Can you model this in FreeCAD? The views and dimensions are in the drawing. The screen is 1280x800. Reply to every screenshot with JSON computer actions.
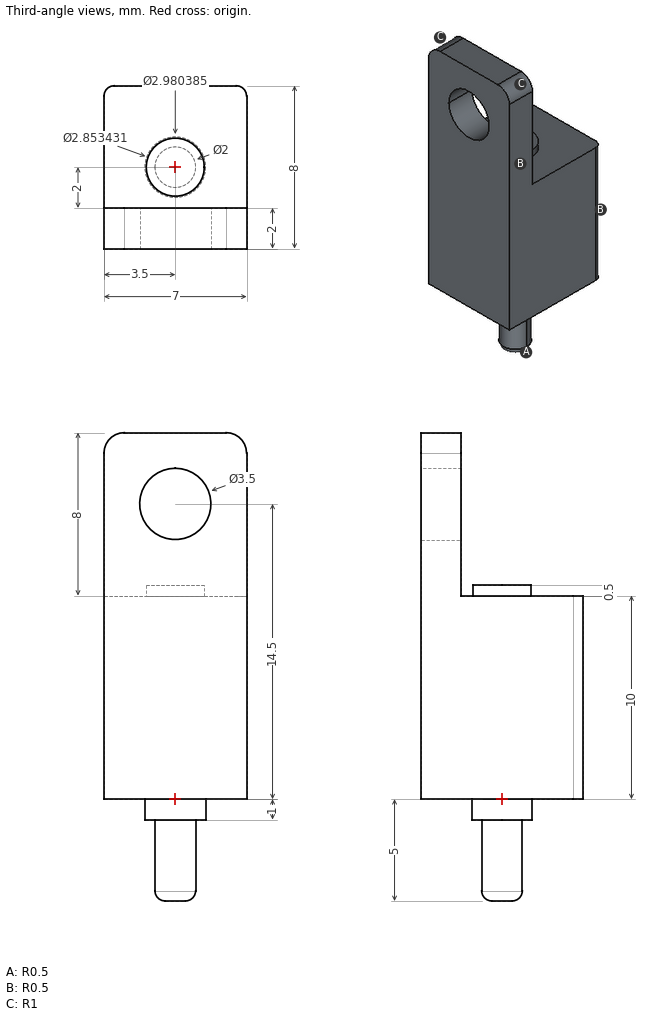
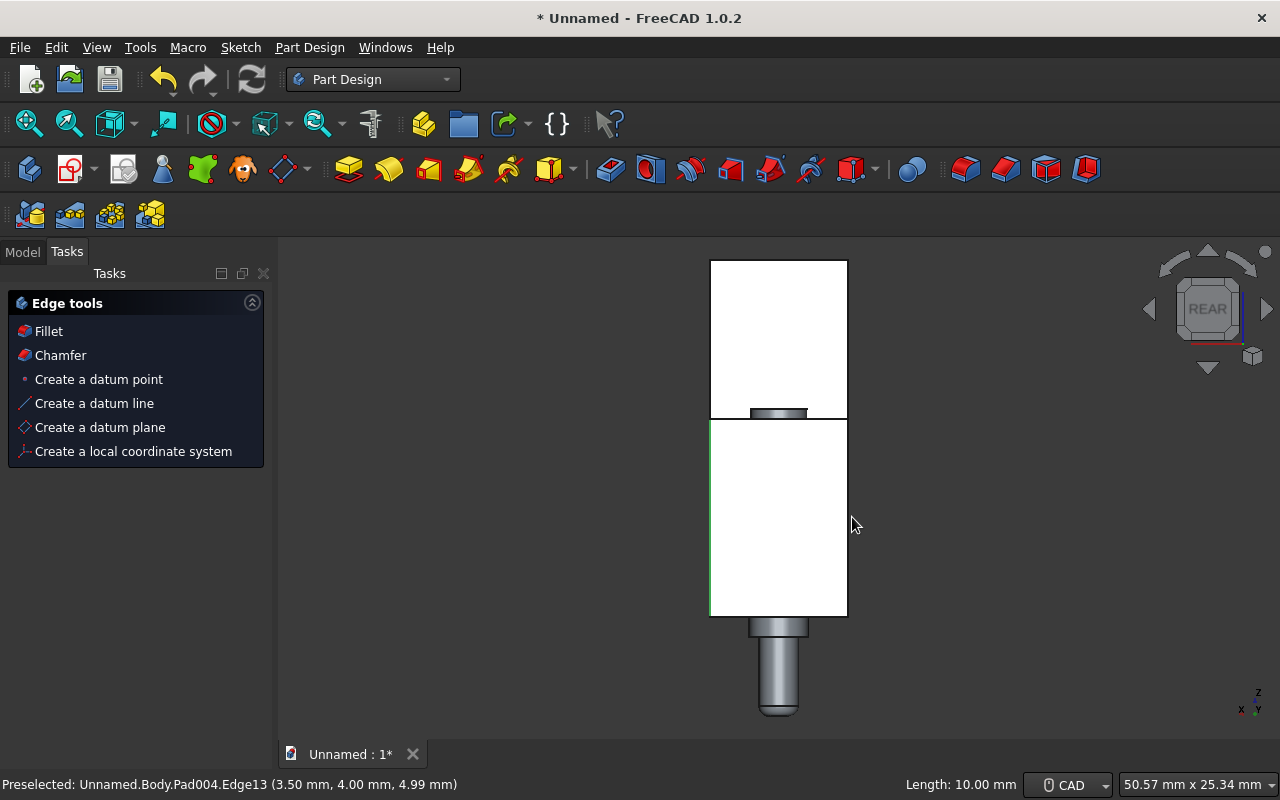
{"action": "left_click", "coordinate": [848, 517], "text": "ctrl"}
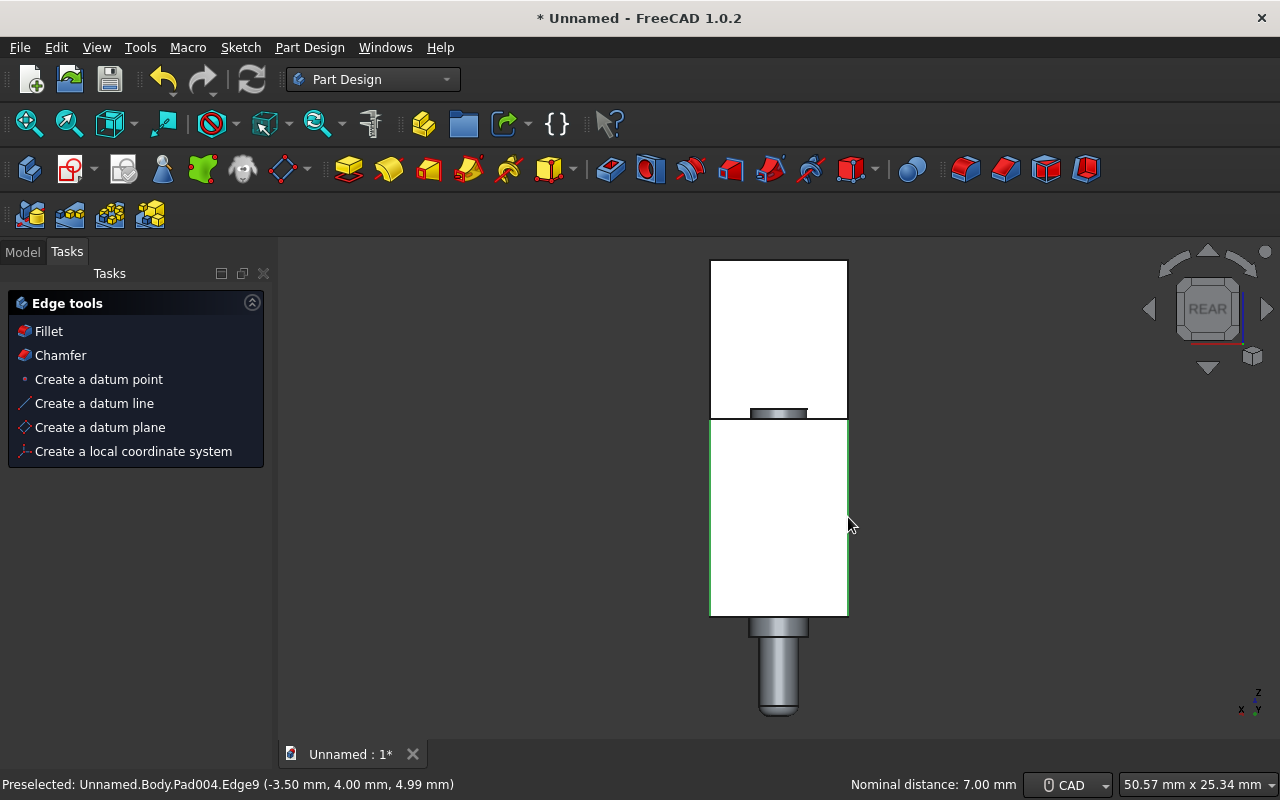
{"action": "left_click", "coordinate": [966, 170]}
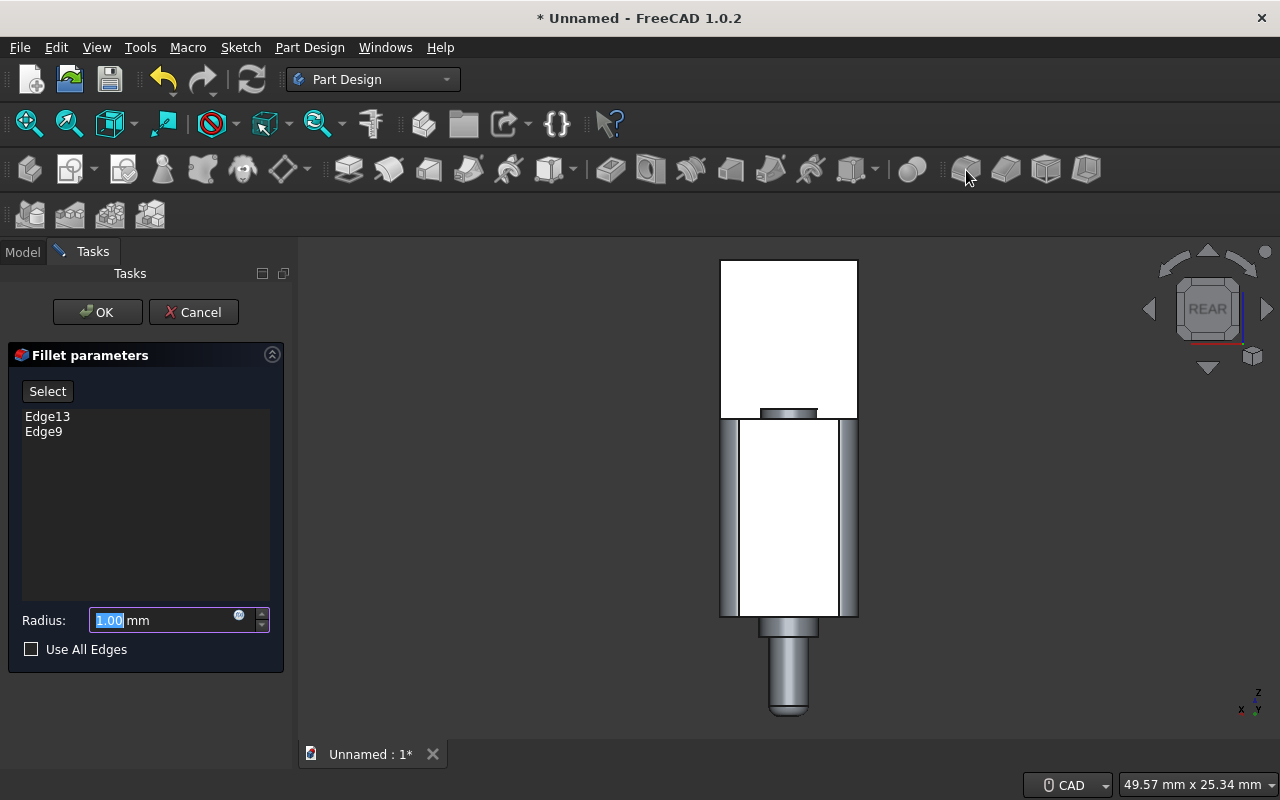
{"action": "type", "text": "0.5"}
{"action": "key", "text": "Tab"}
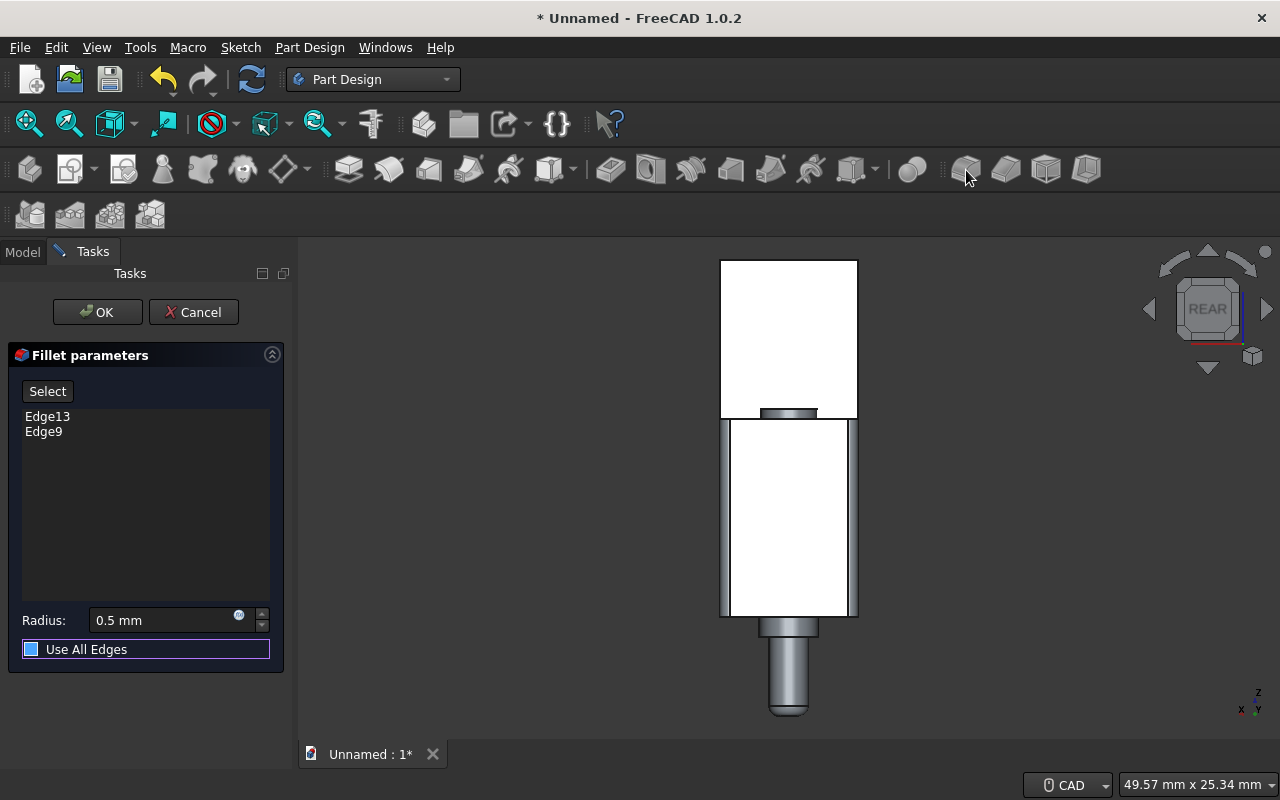
{"action": "left_click", "coordinate": [98, 312]}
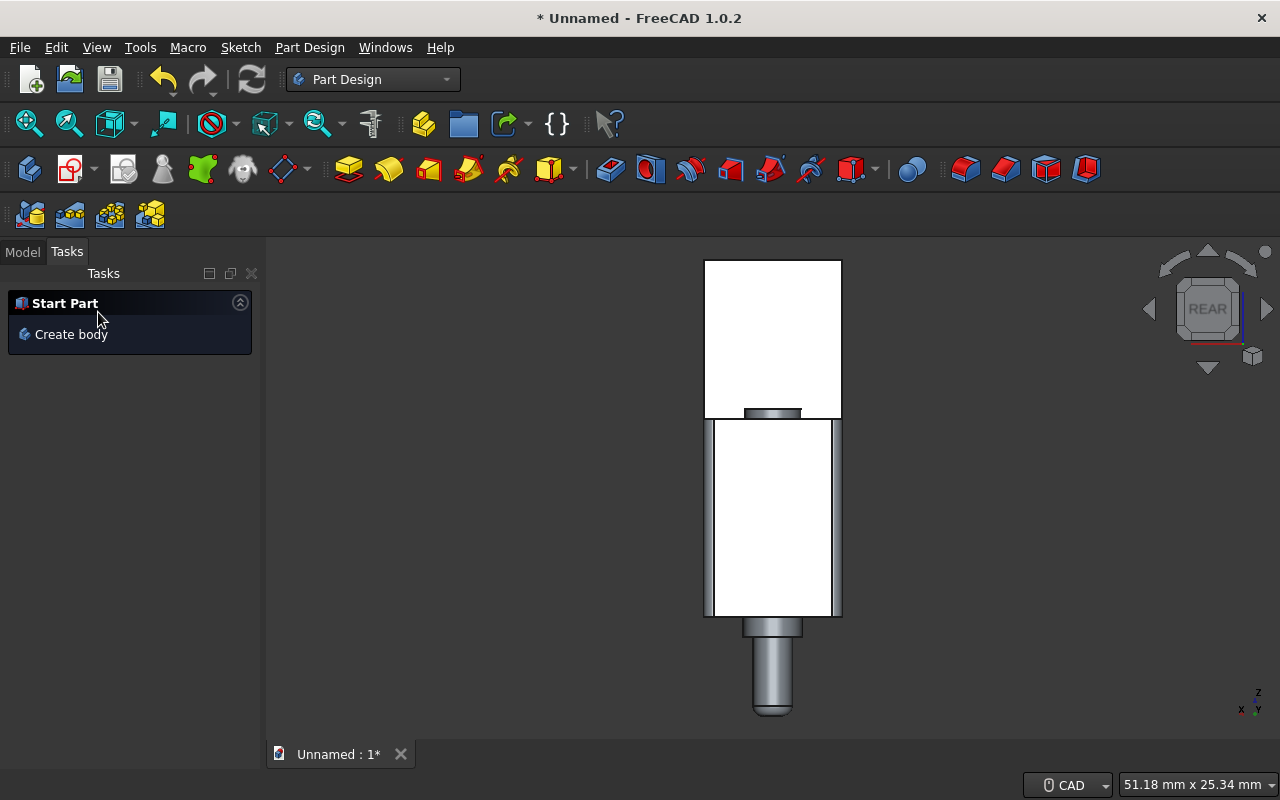
{"action": "key", "text": "0"}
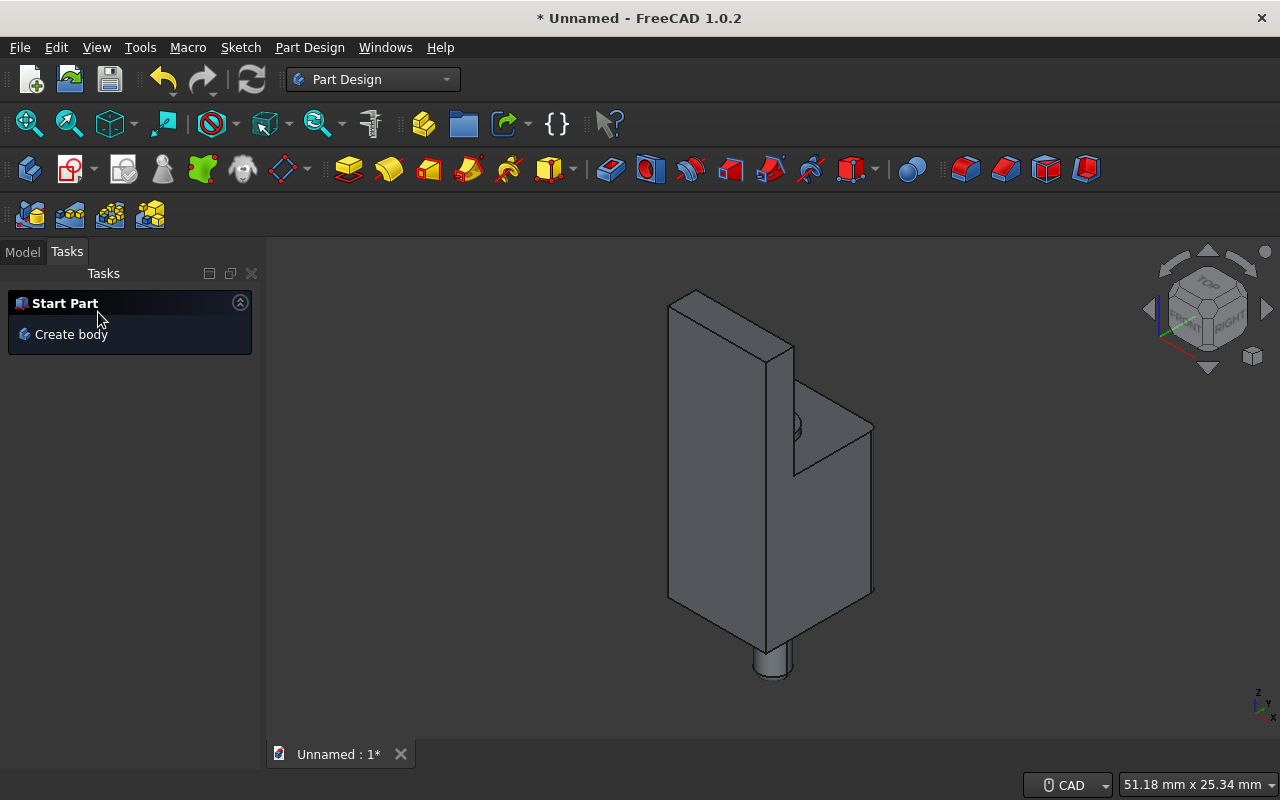
{"action": "left_click", "coordinate": [780, 354]}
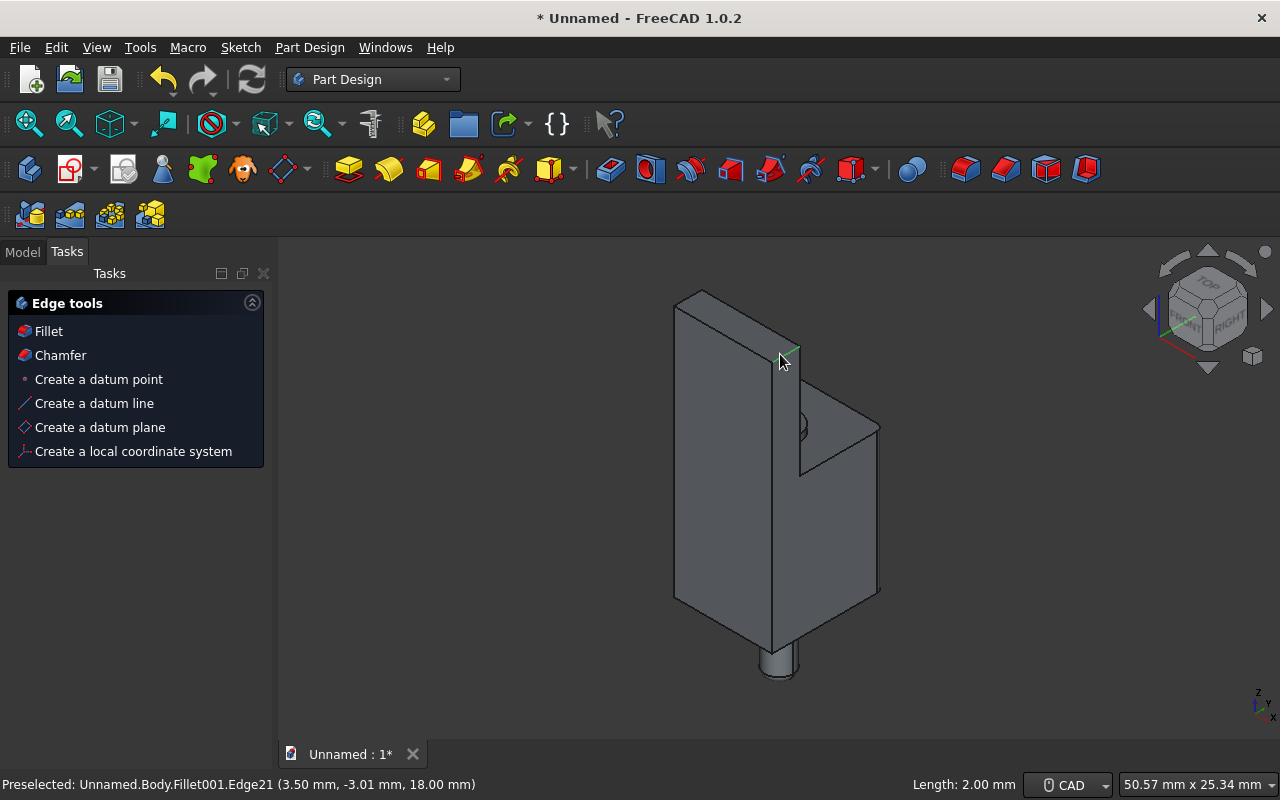
{"action": "key", "text": "2"}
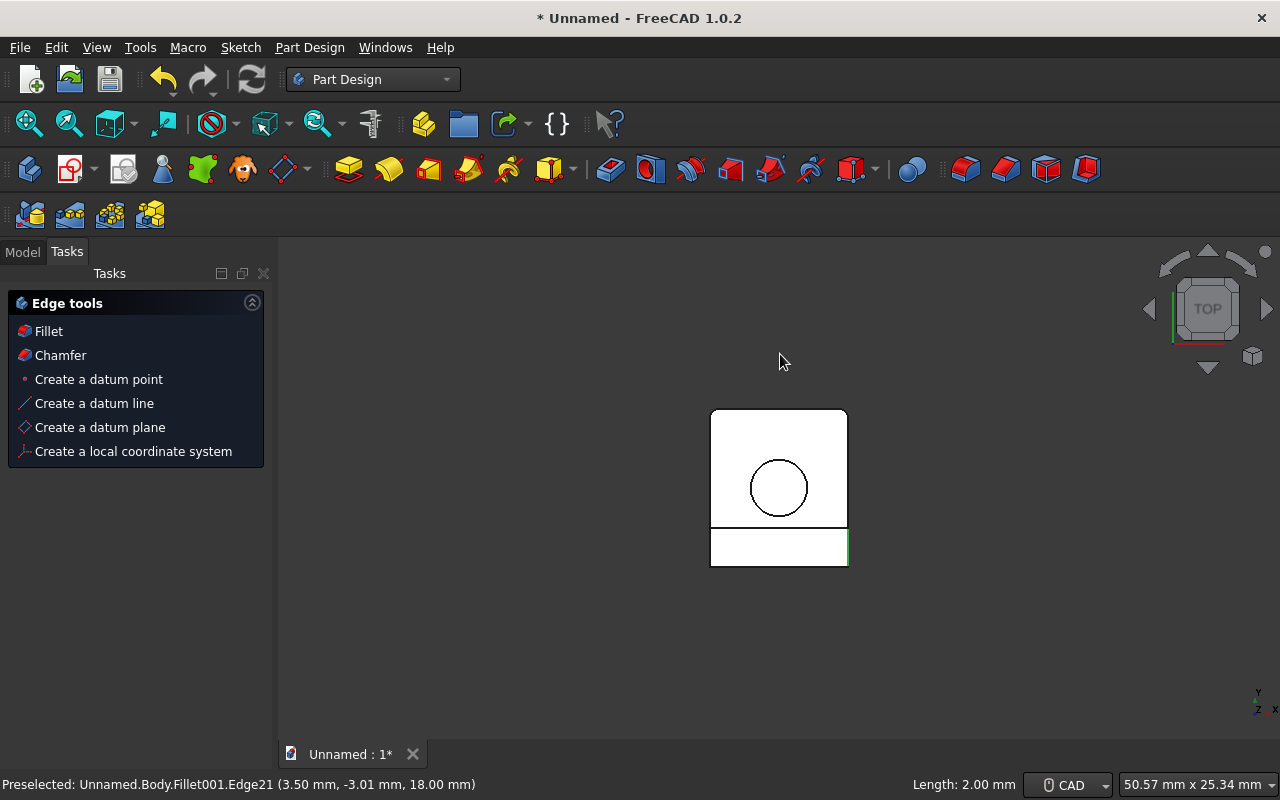
{"action": "key", "text": "v f"}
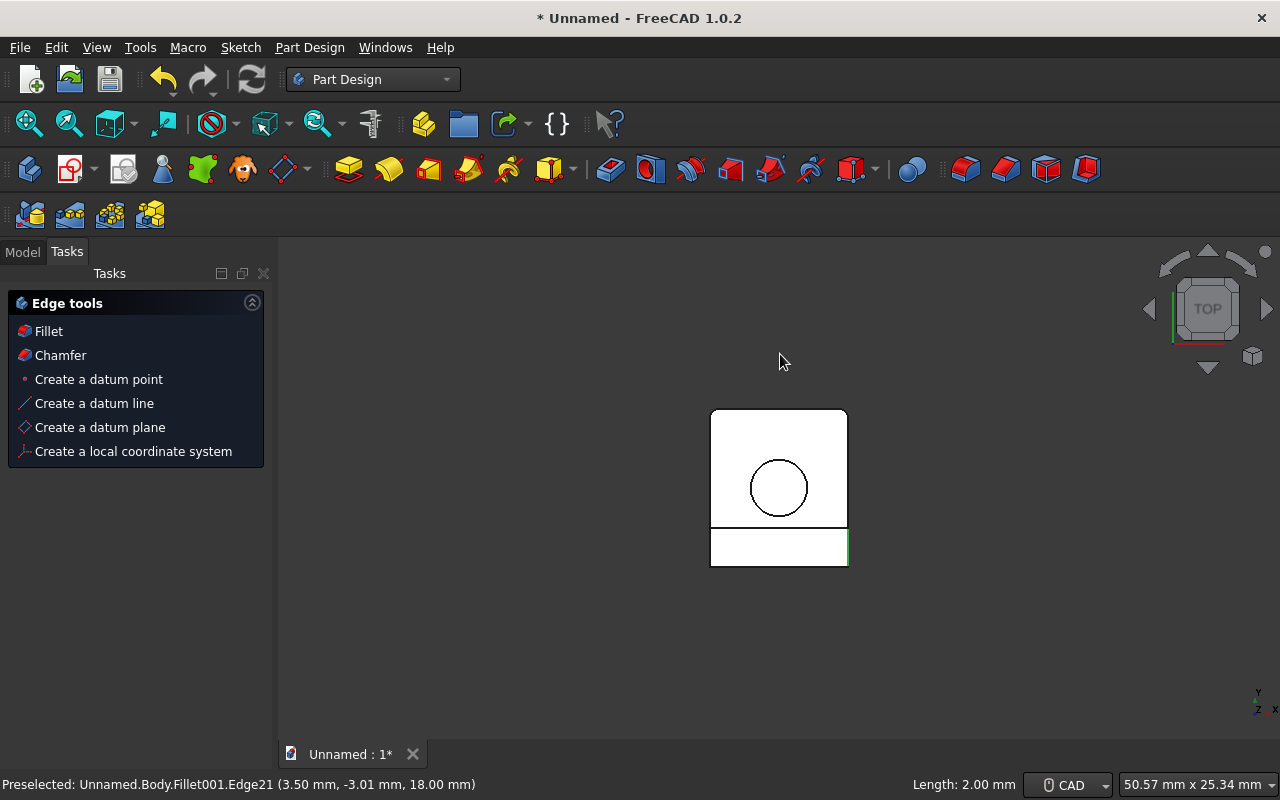
{"action": "left_click", "coordinate": [710, 546], "text": "ctrl"}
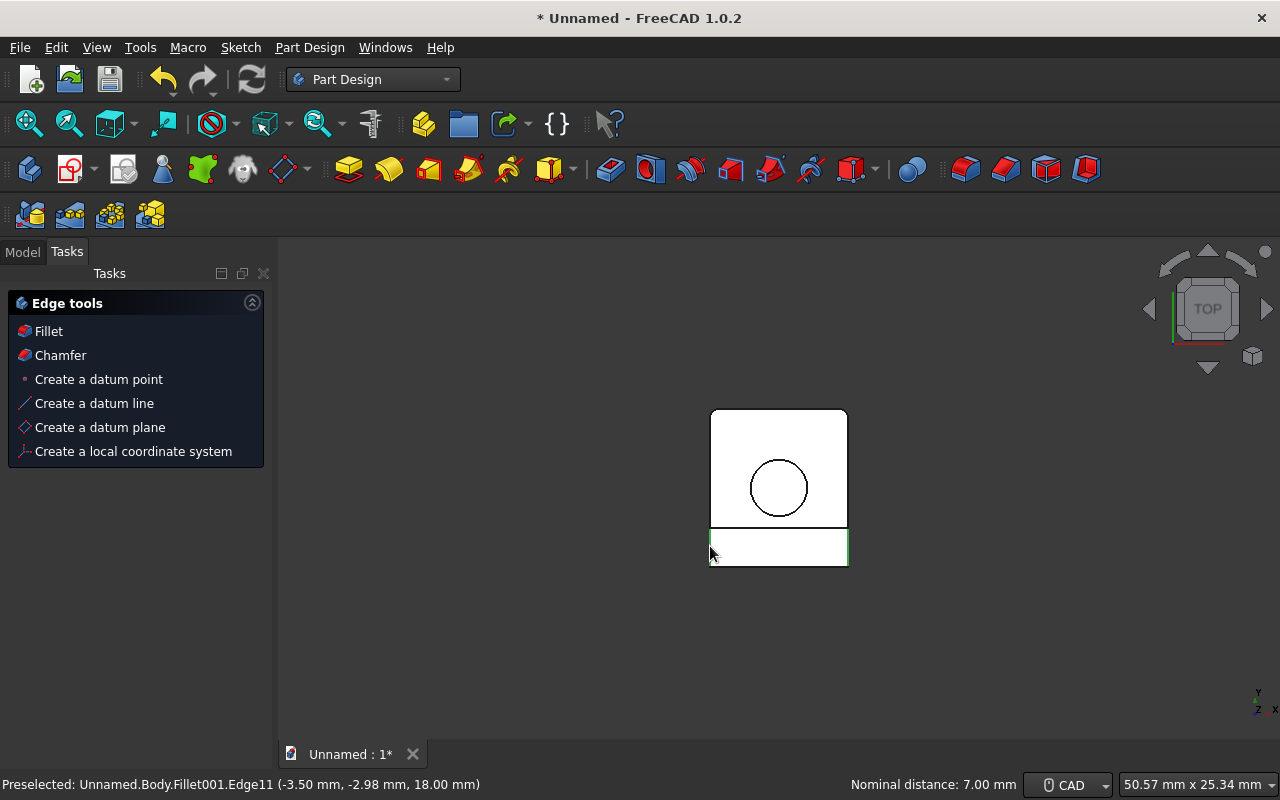
{"action": "left_click", "coordinate": [966, 170]}